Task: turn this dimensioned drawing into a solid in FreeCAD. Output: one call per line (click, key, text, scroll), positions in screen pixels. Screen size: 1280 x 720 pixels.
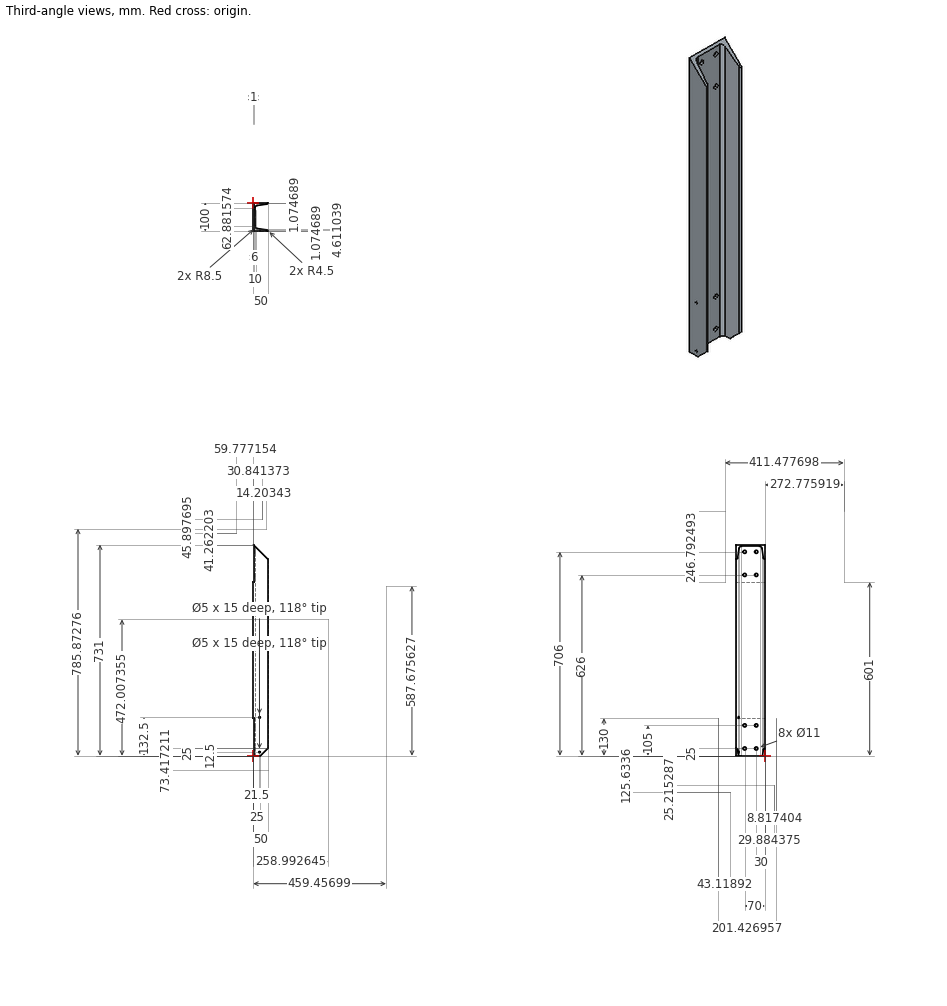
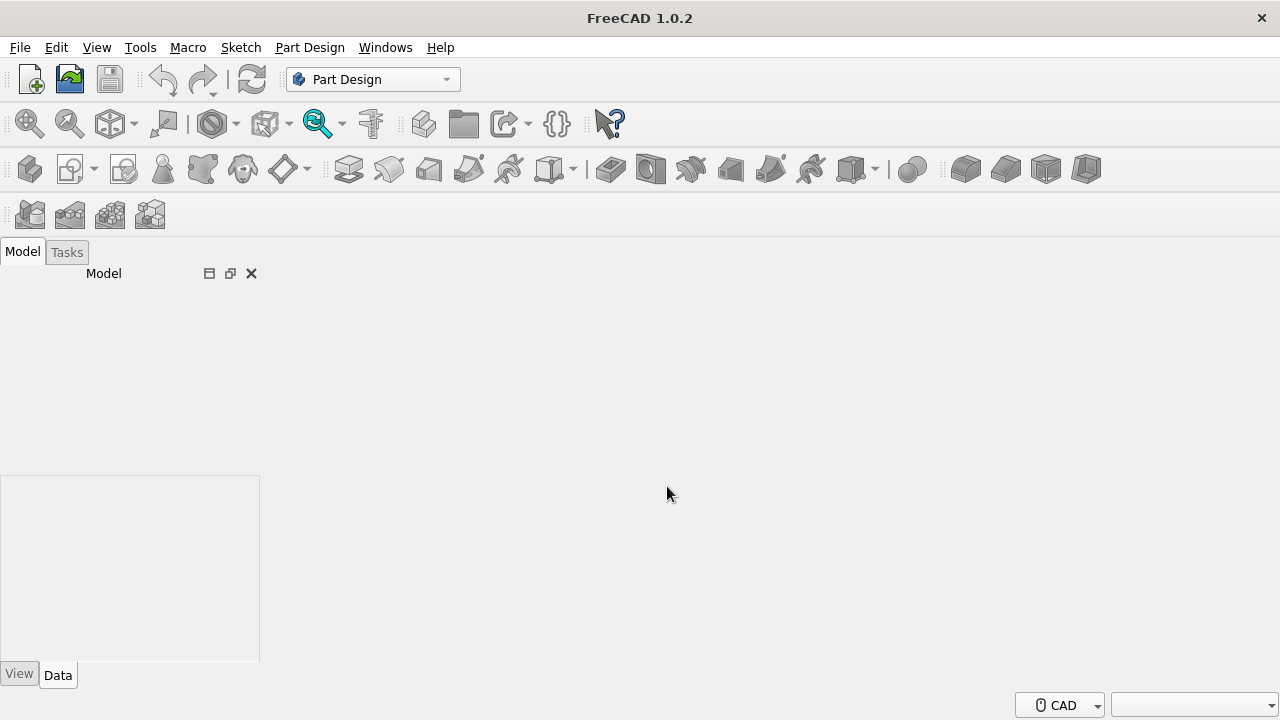
key(ctrl+n)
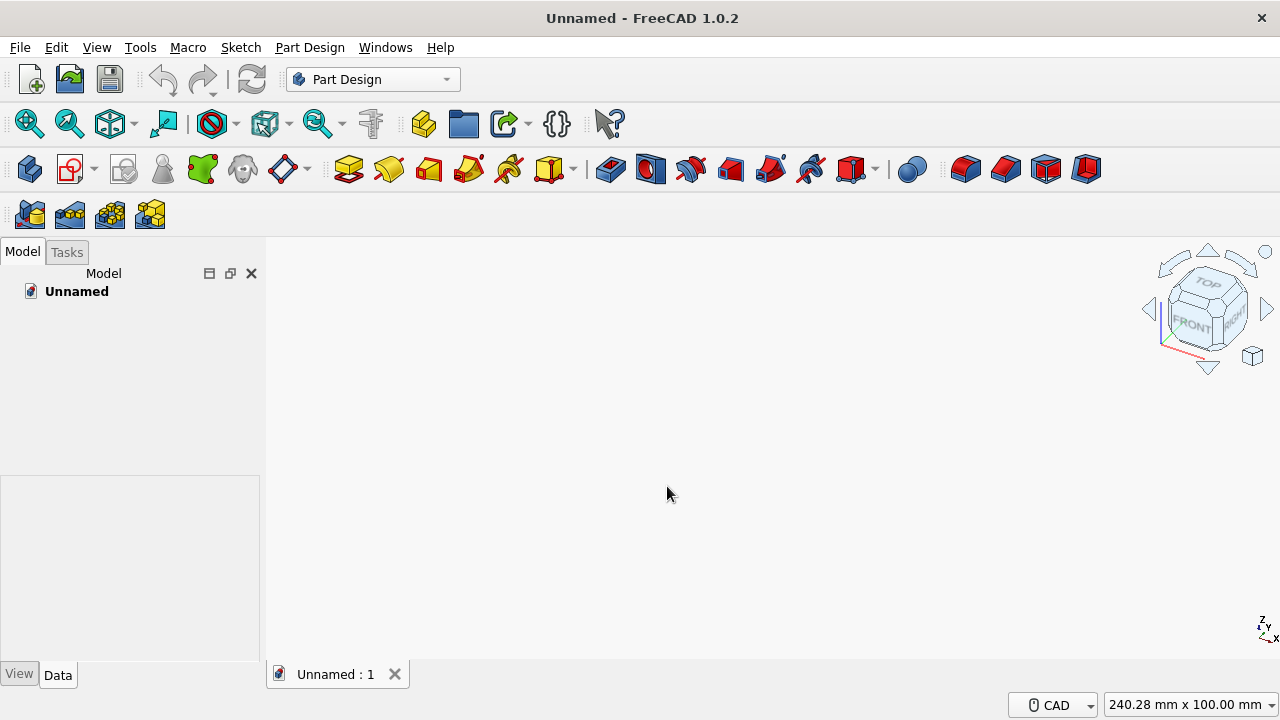
click(70, 170)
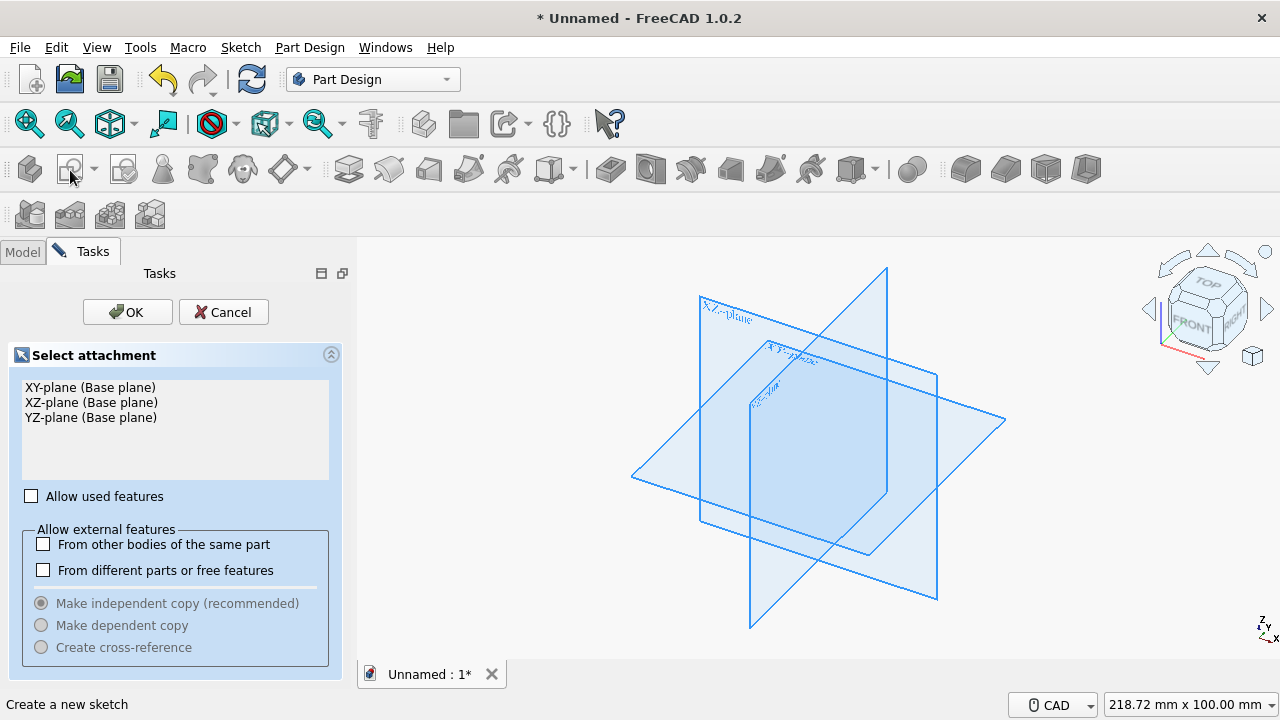
click(82, 388)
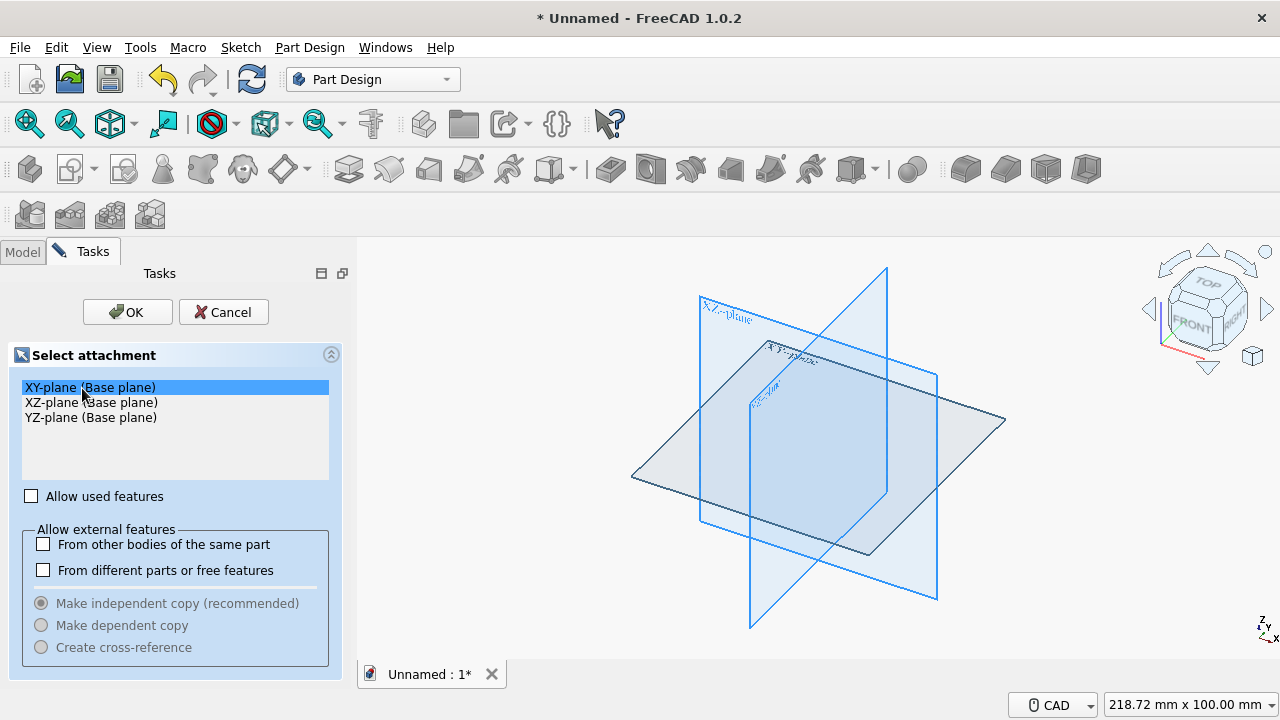
click(128, 312)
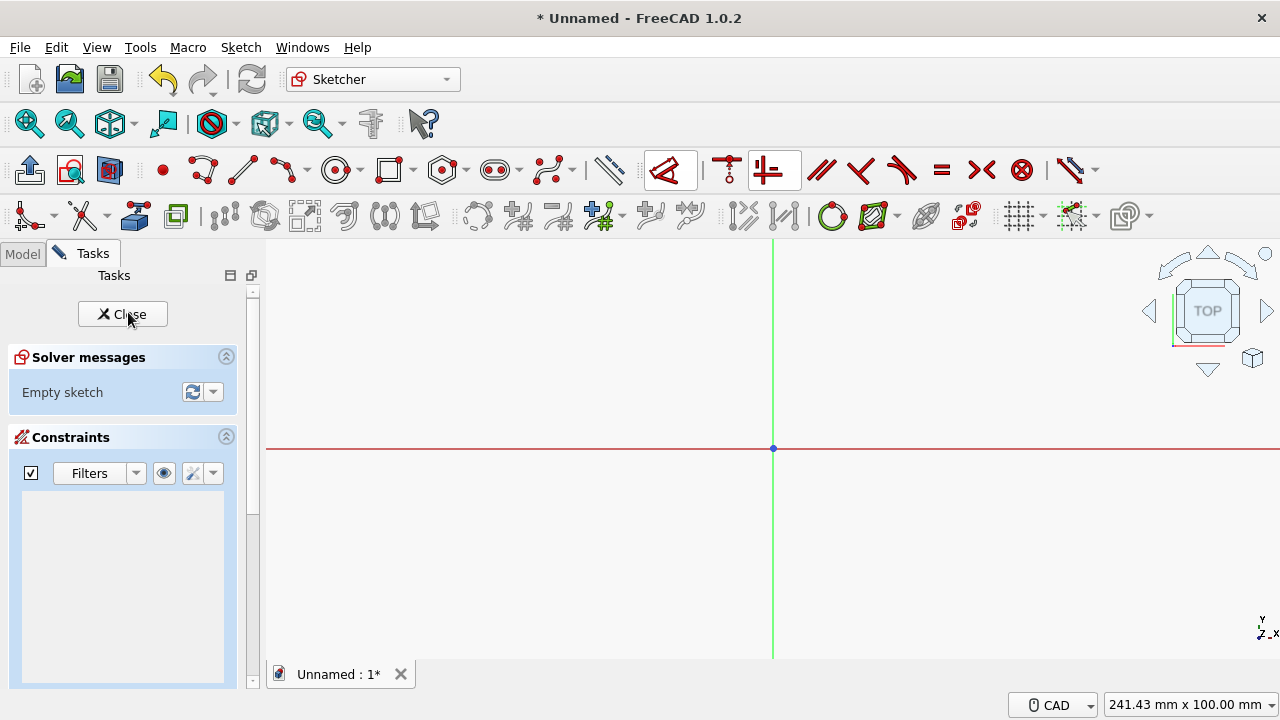
scroll(493, 267, down, 3)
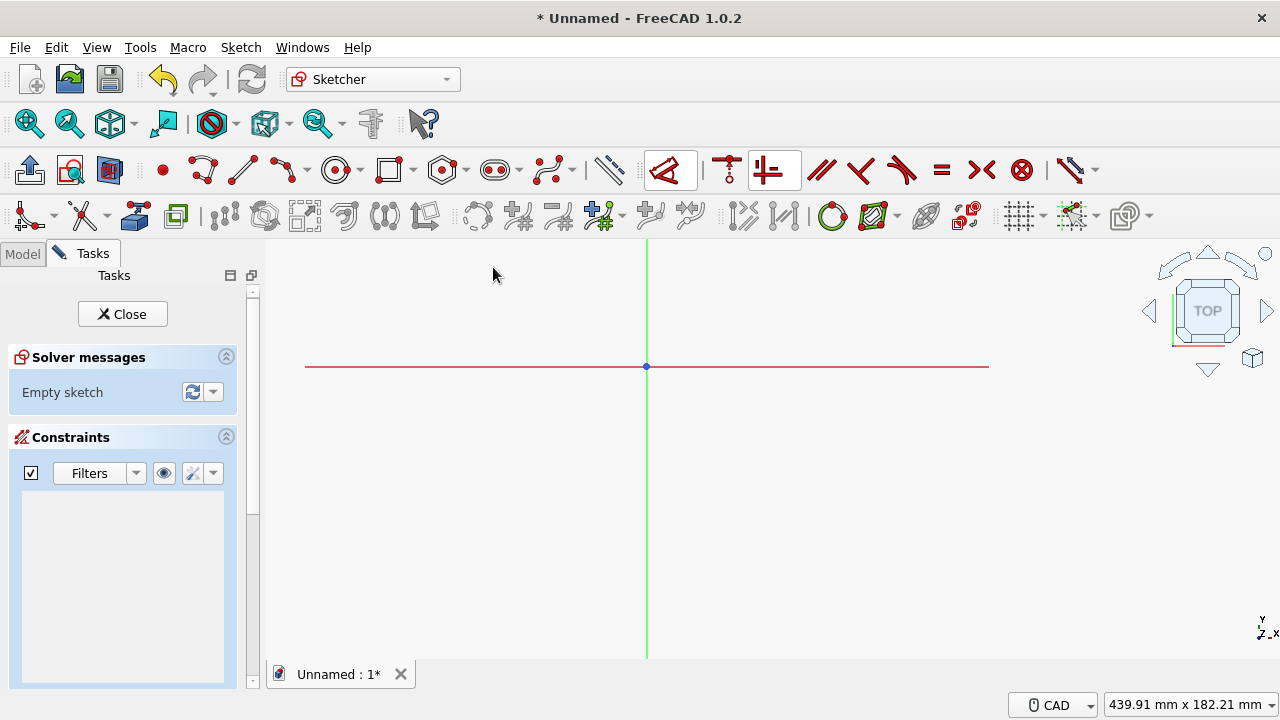
click(244, 170)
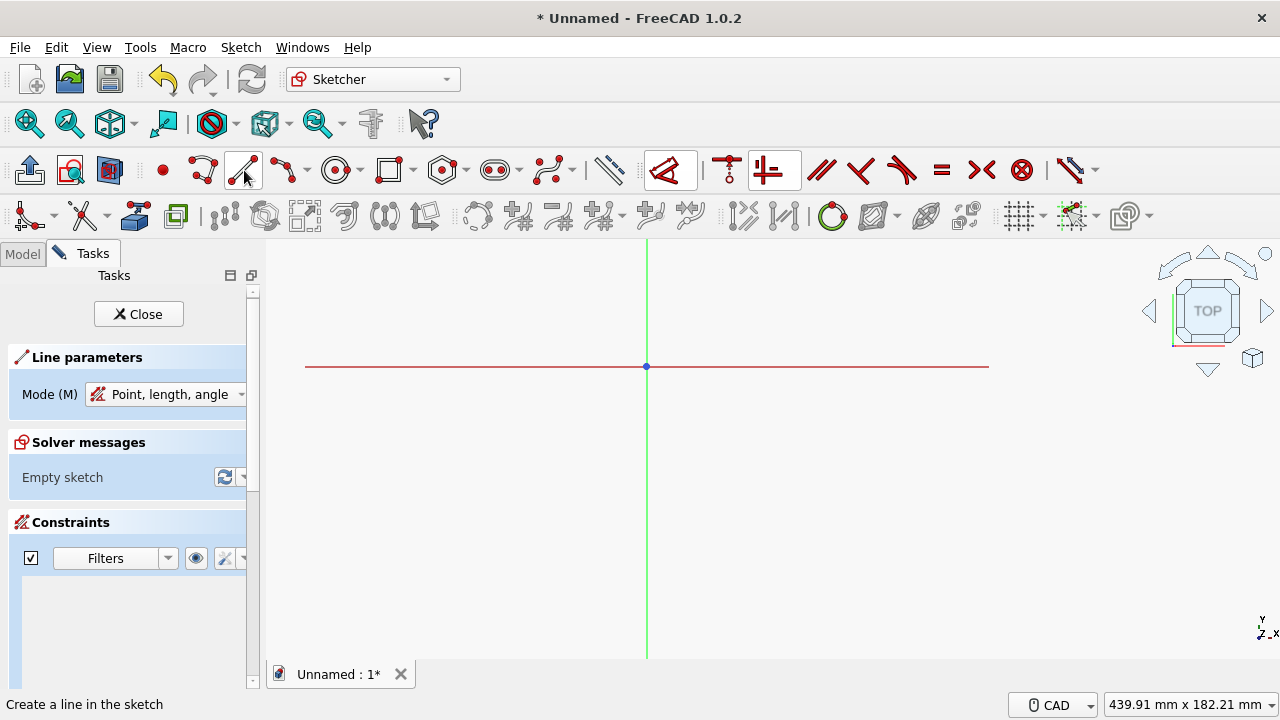
click(753, 585)
click(677, 574)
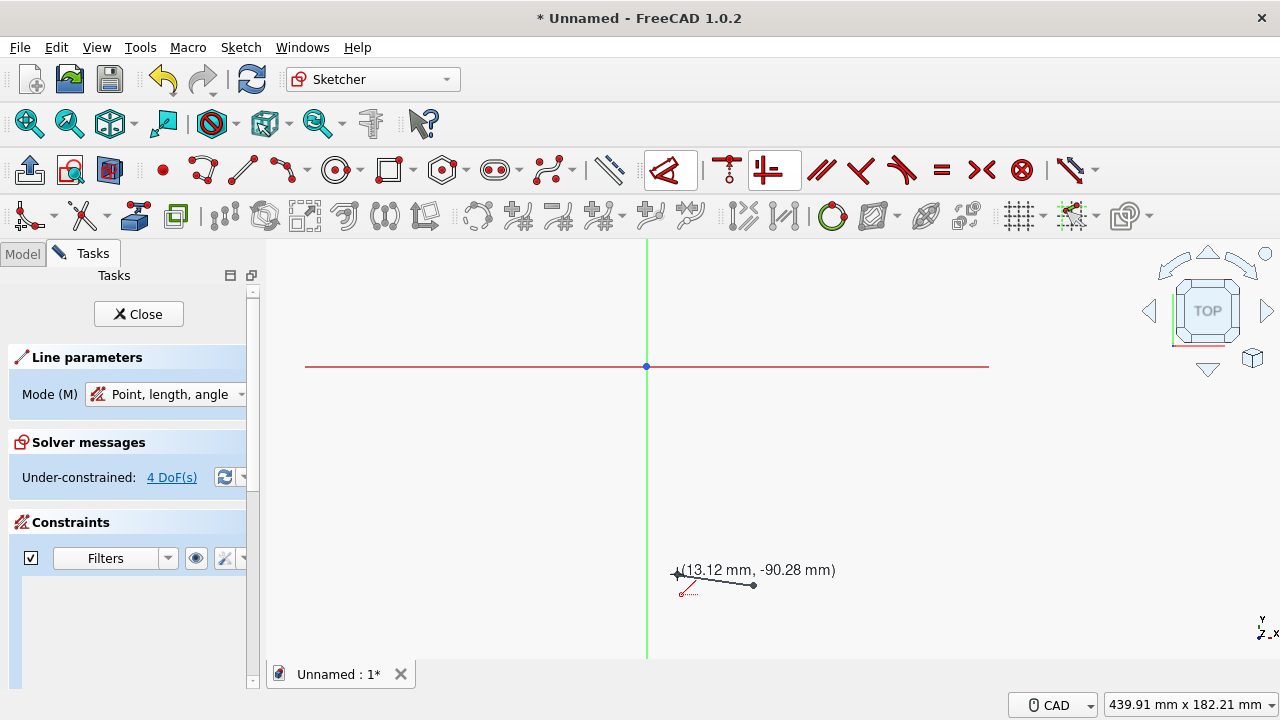
click(661, 555)
click(661, 410)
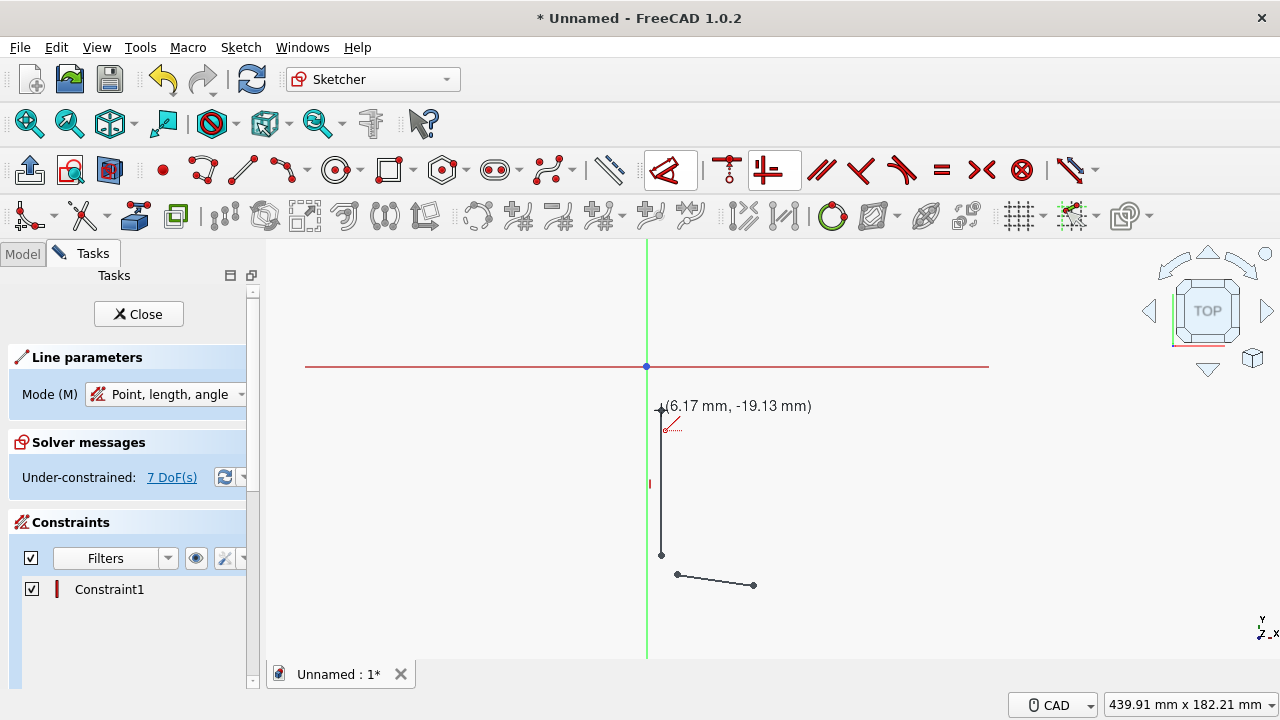
click(677, 390)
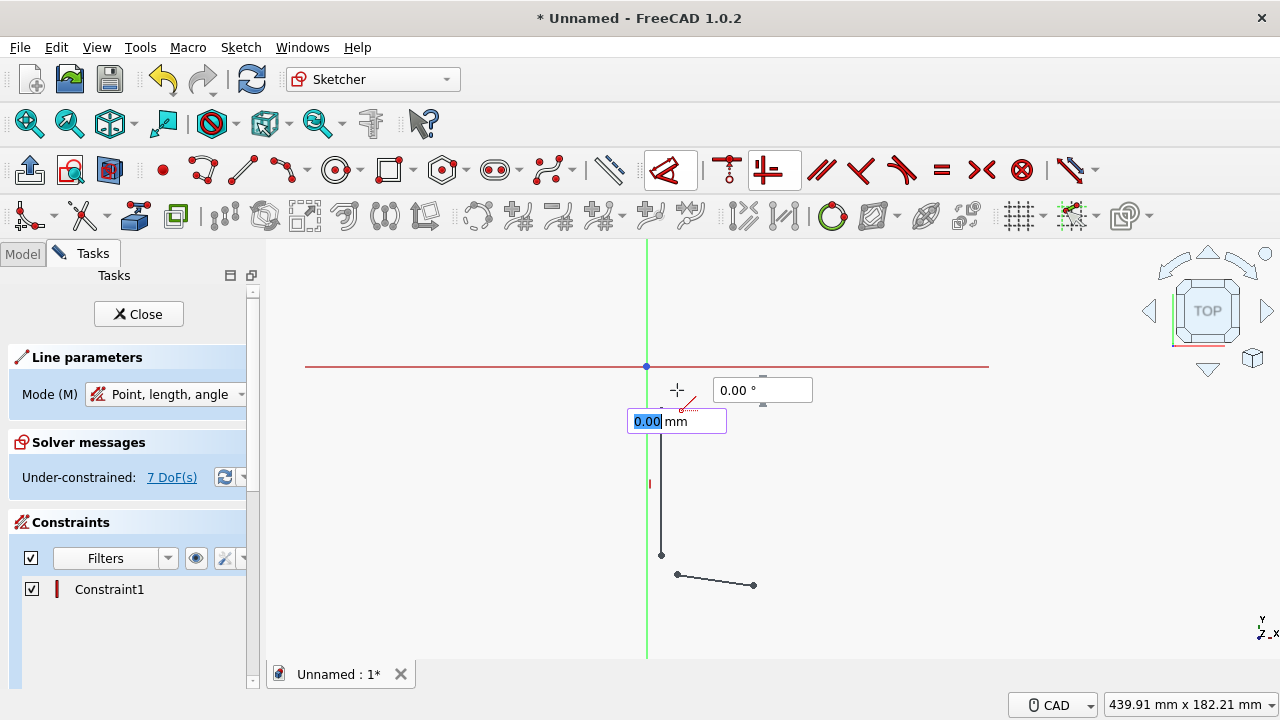
scroll(753, 380, up, 2)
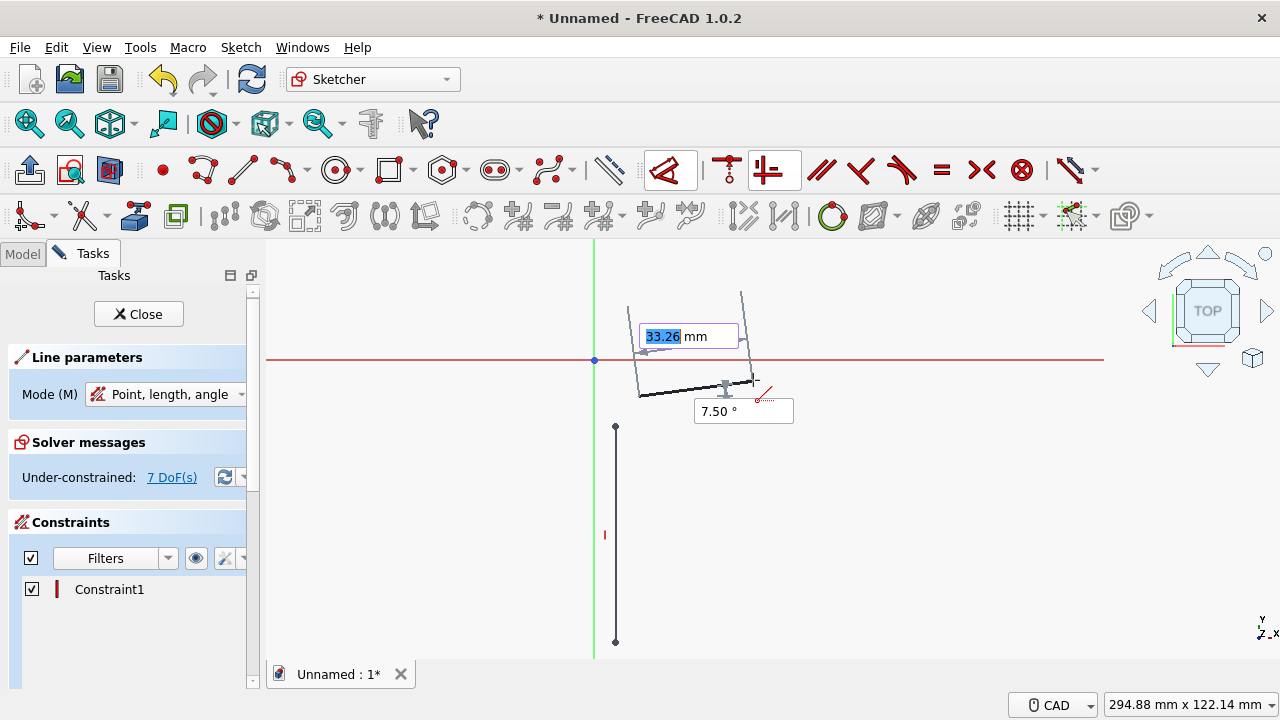
click(753, 379)